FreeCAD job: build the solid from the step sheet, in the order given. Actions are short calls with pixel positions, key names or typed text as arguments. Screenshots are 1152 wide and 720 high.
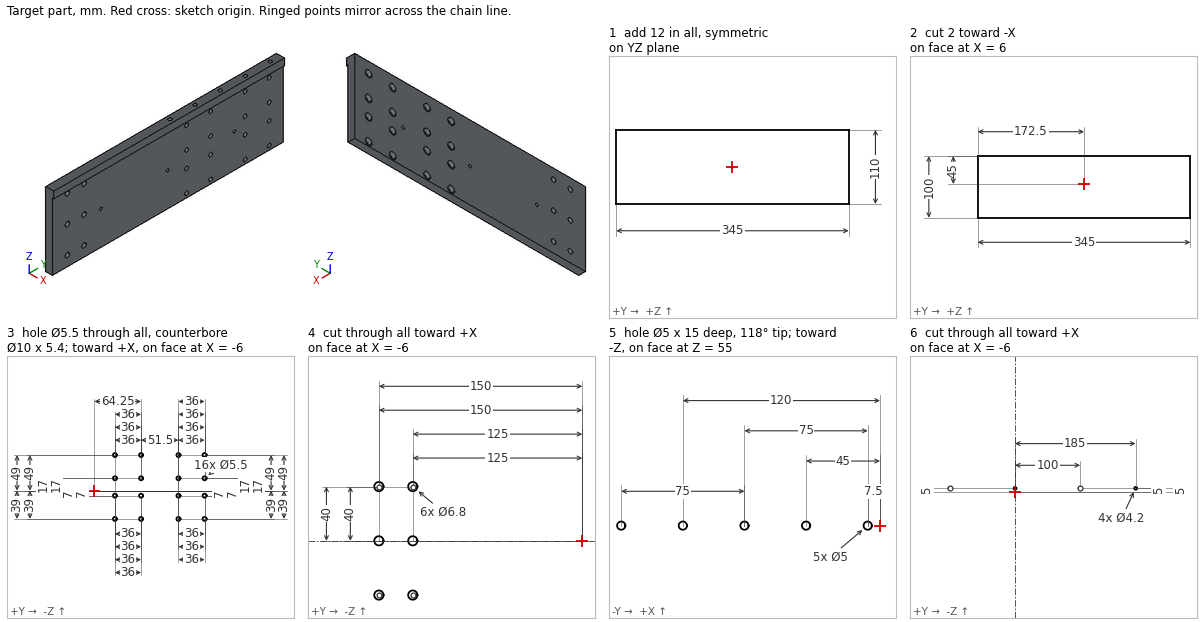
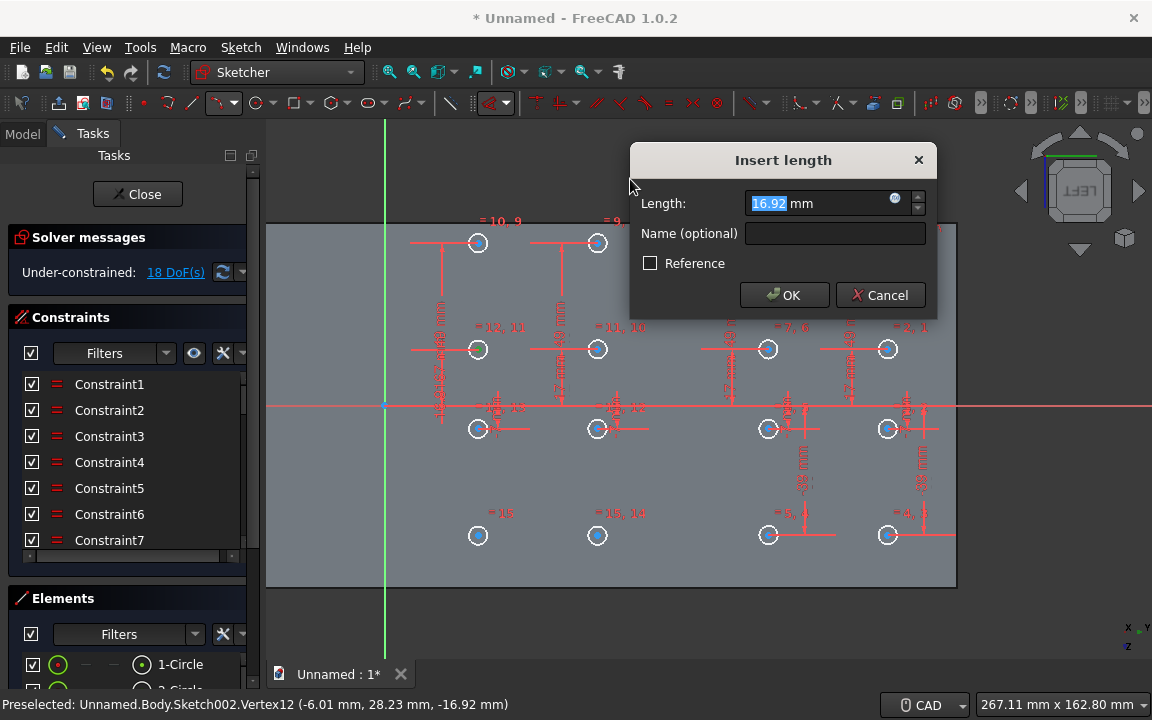
text(17)
key(Return)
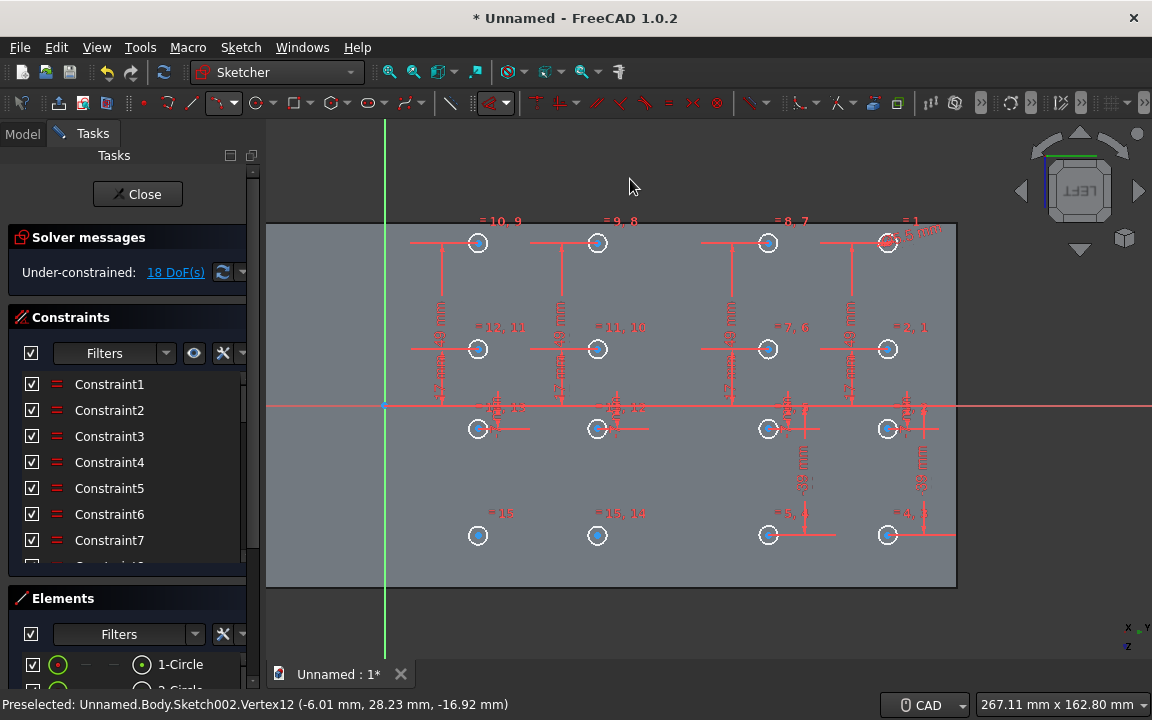
click(598, 536)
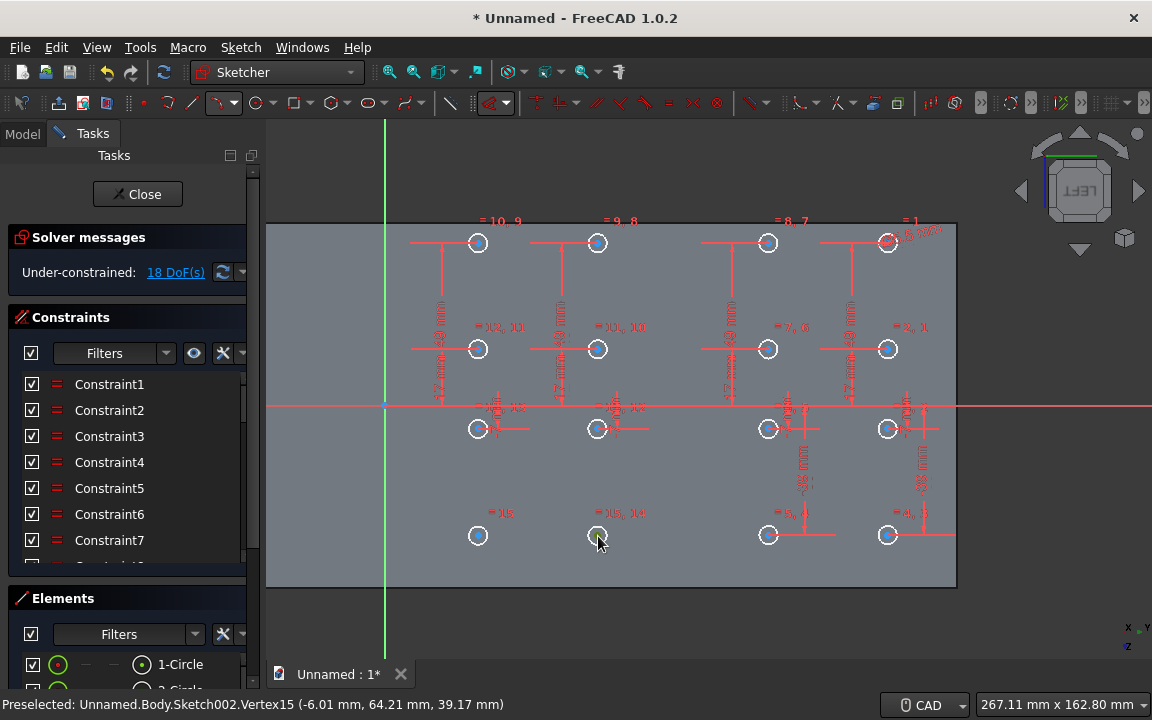
key(i)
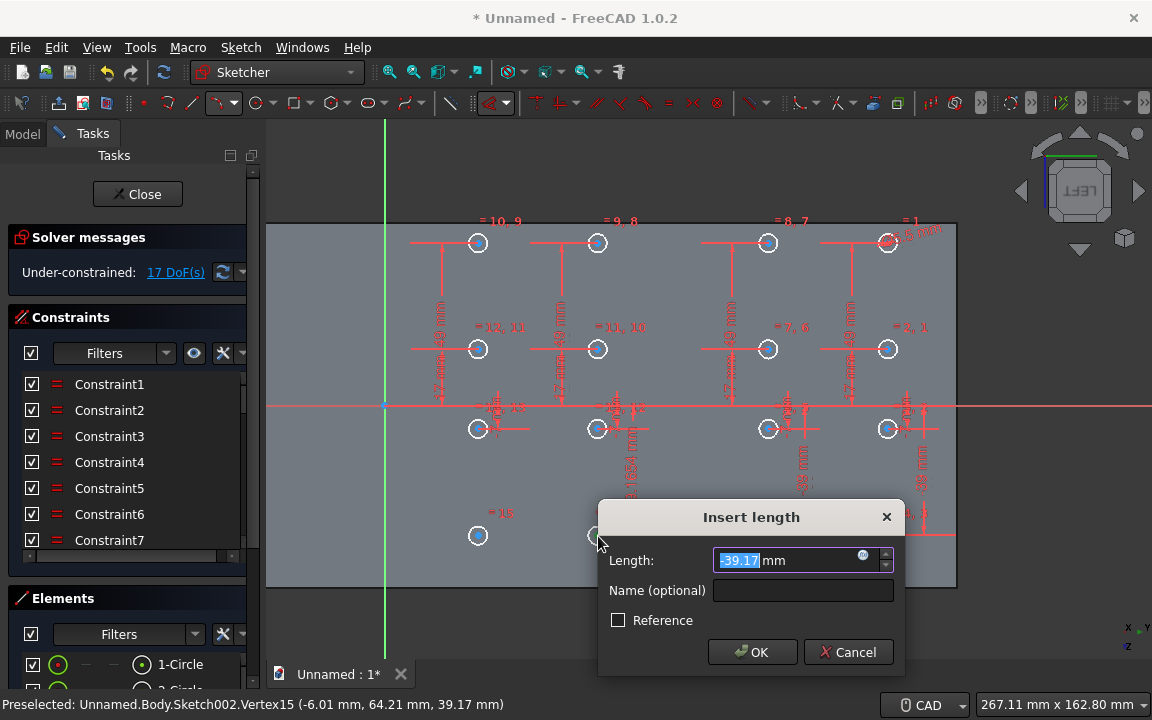
text(-39)
key(Return)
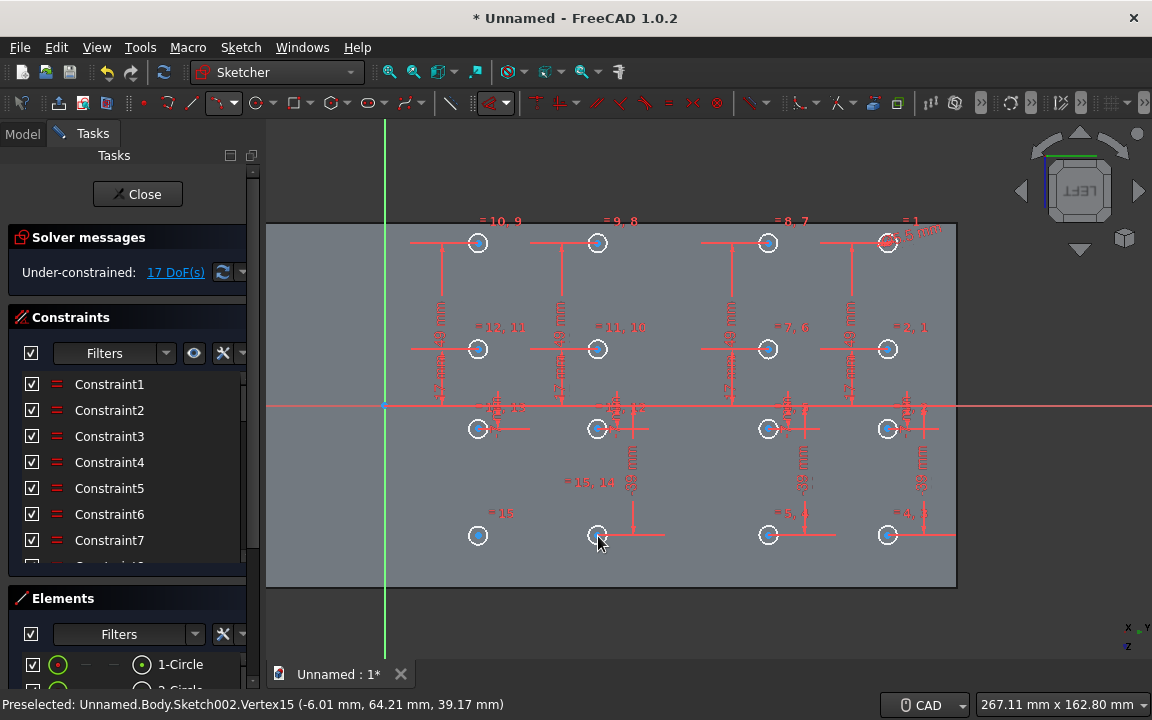
click(478, 536)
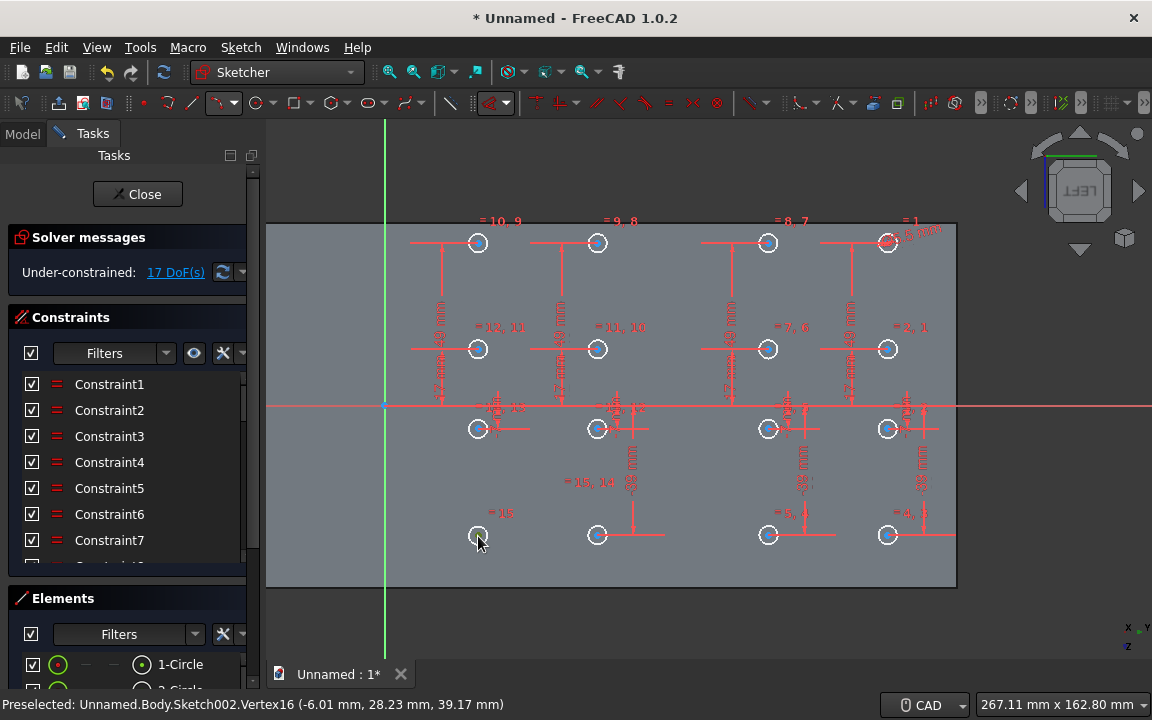
click(508, 104)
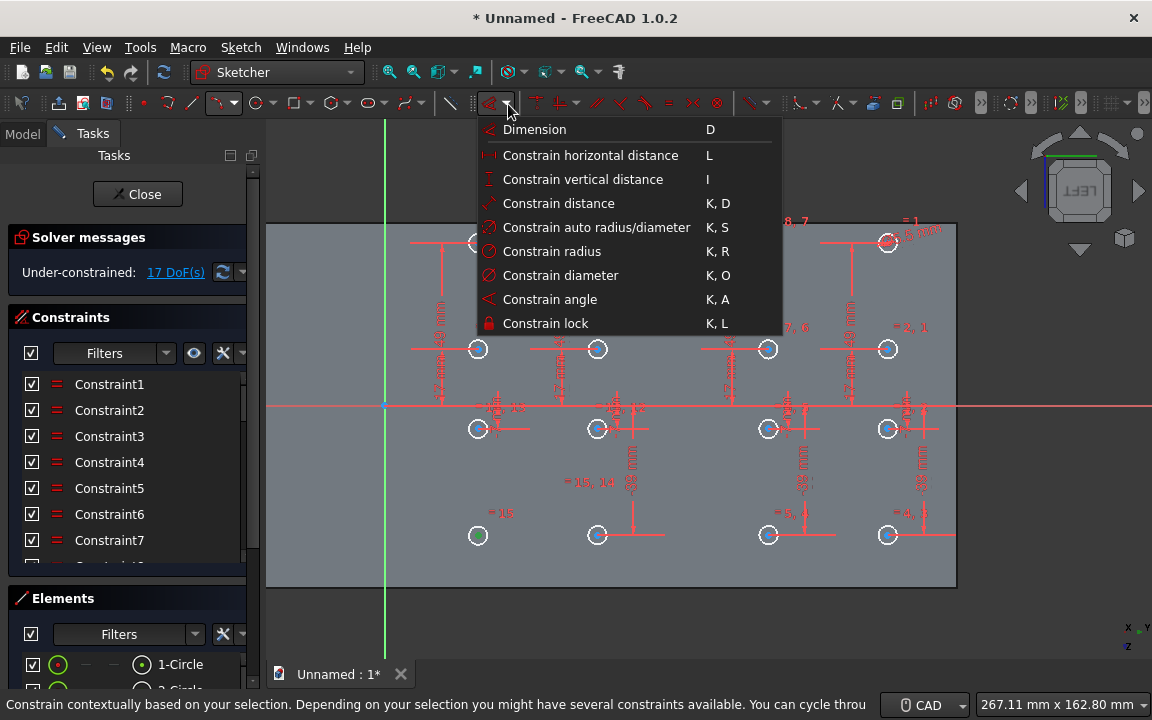
click(630, 179)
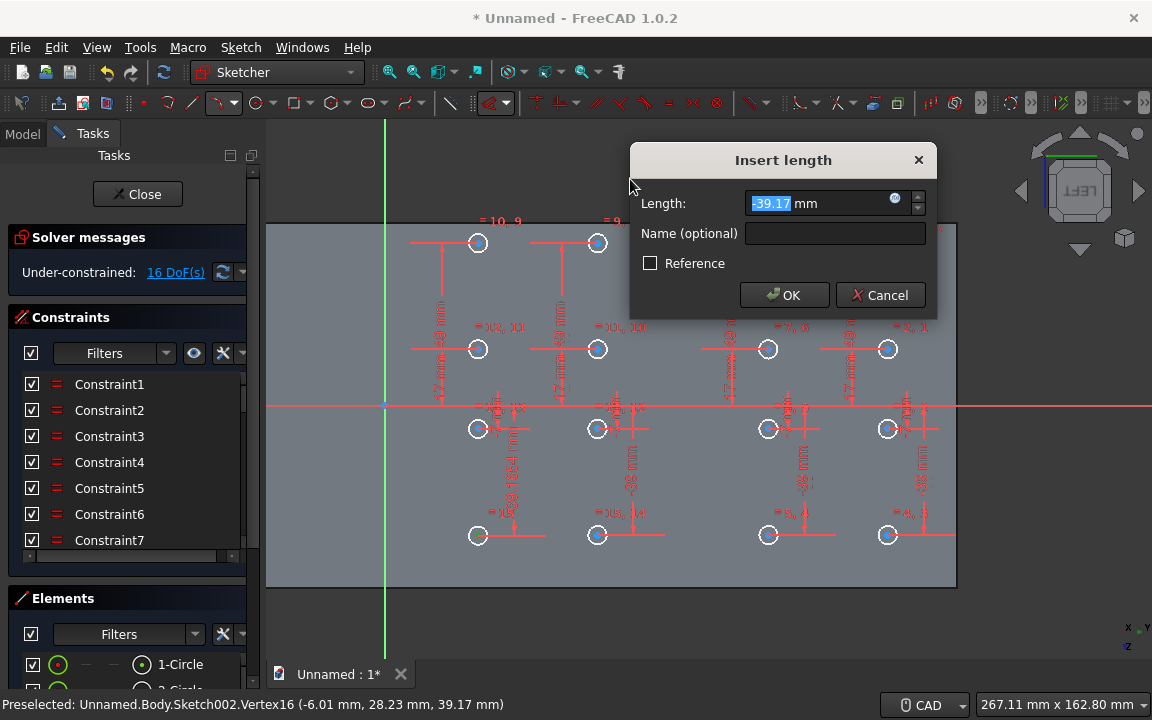
text(-39)
key(Return)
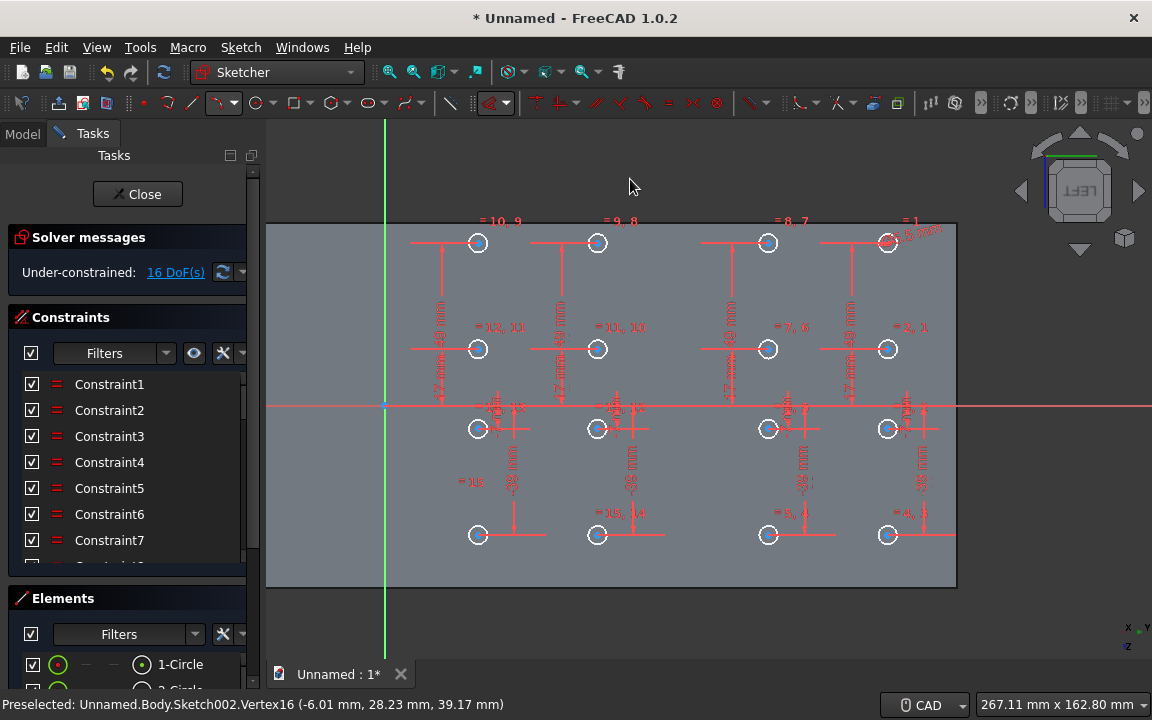
click(888, 535)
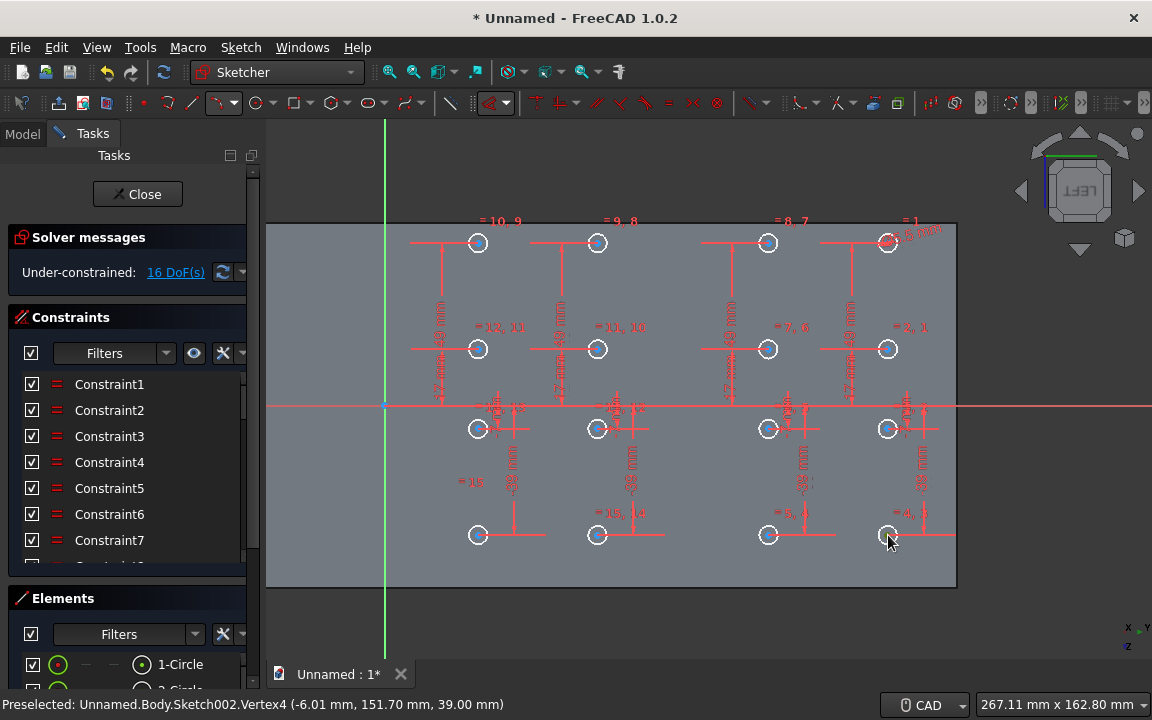
click(769, 535)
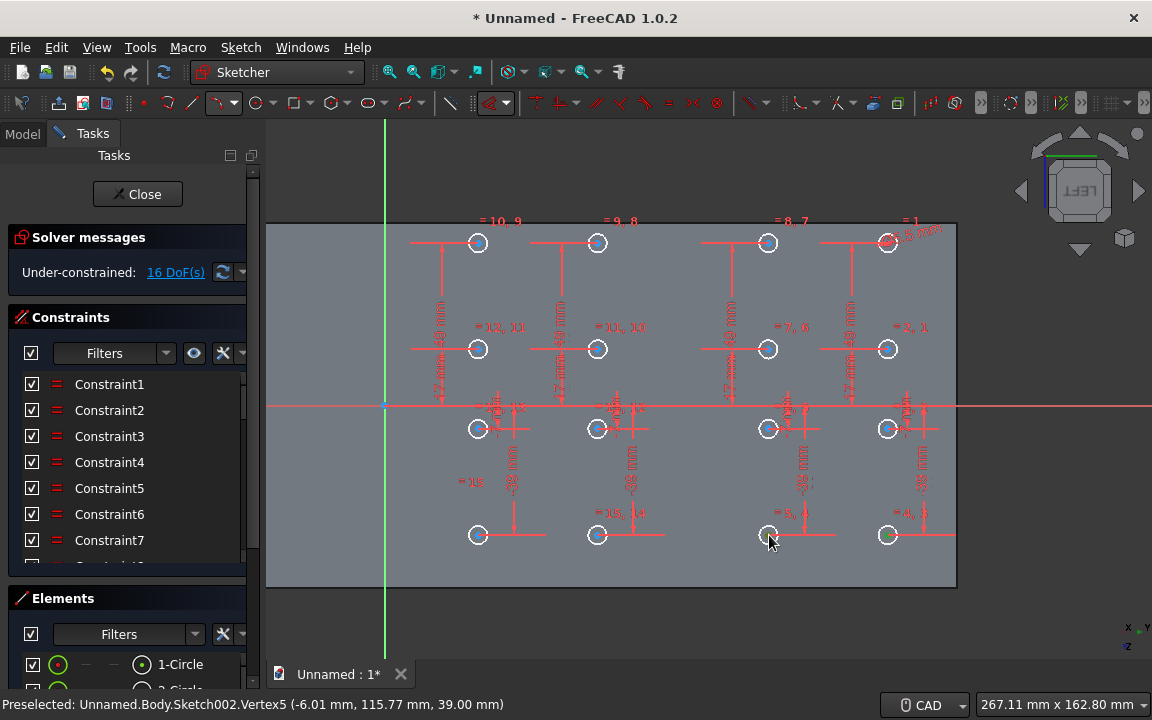
click(508, 104)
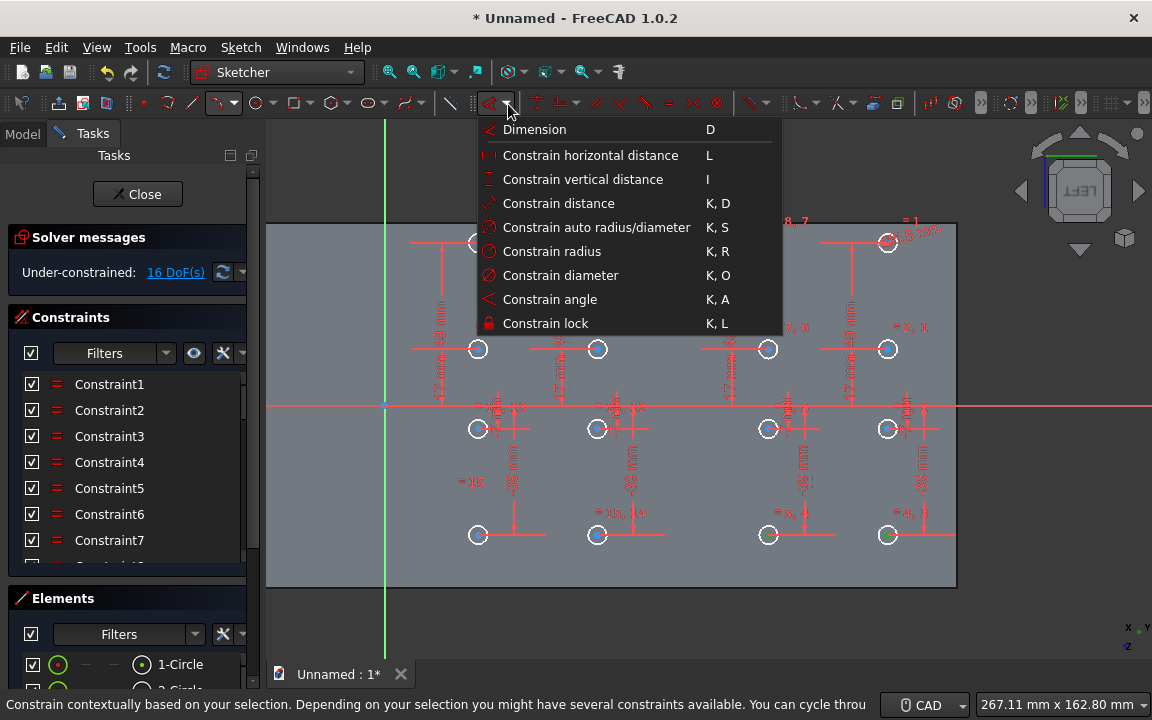
click(630, 155)